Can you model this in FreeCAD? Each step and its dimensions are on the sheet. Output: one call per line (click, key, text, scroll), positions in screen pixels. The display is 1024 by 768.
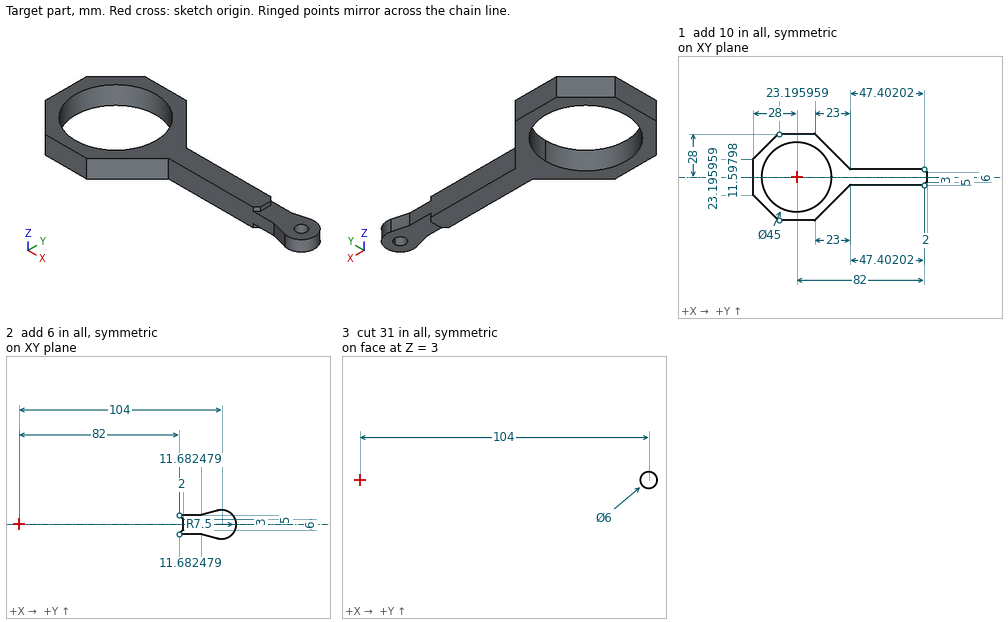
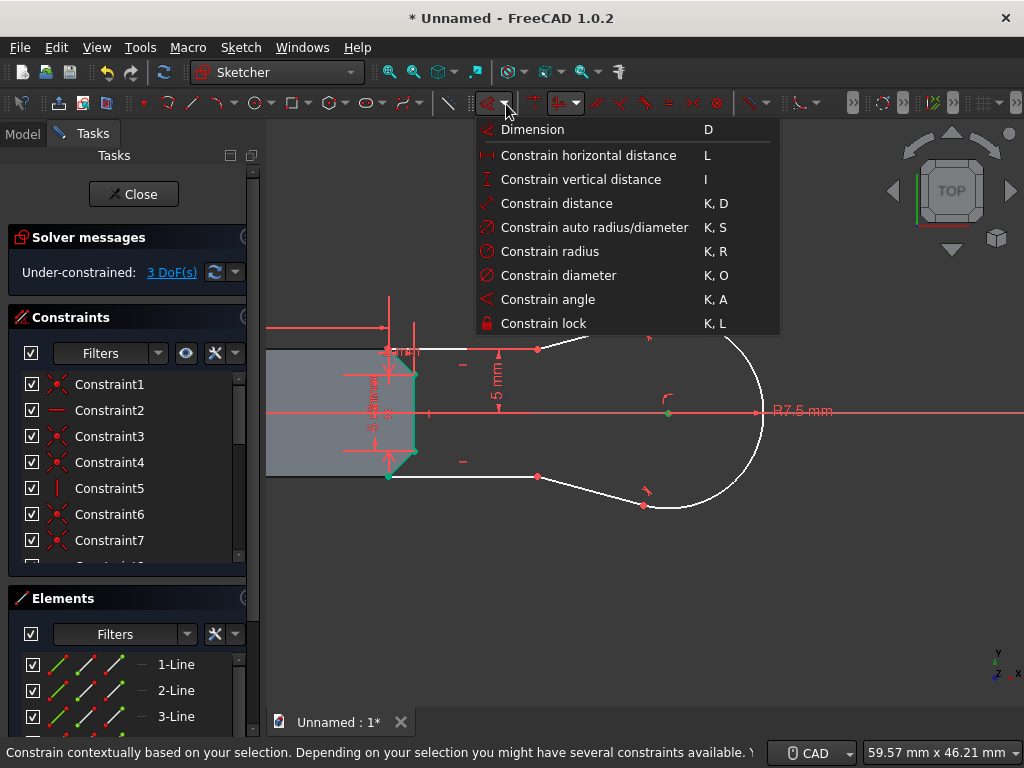
click(628, 155)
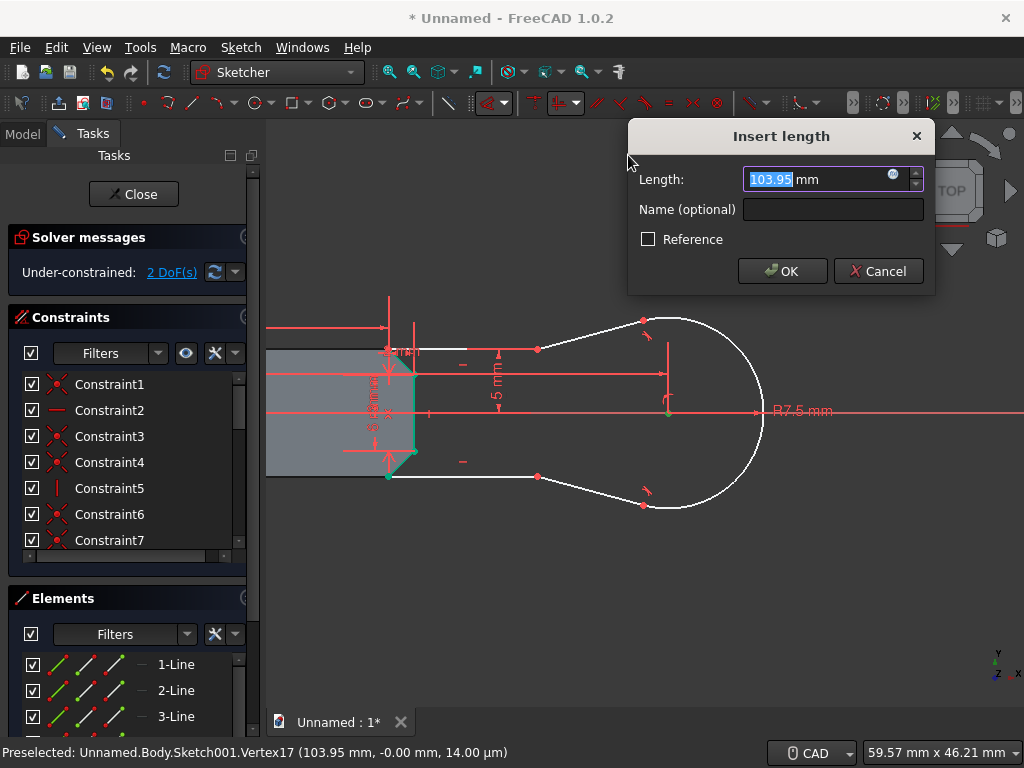
text(104)
key(Return)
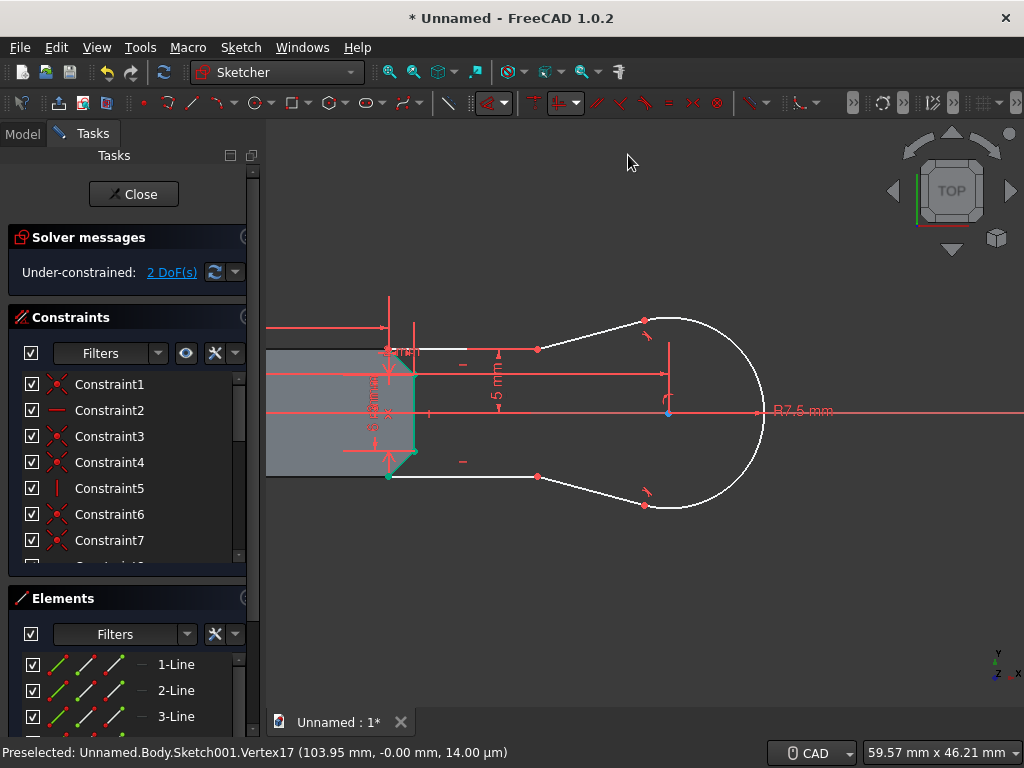
click(493, 349)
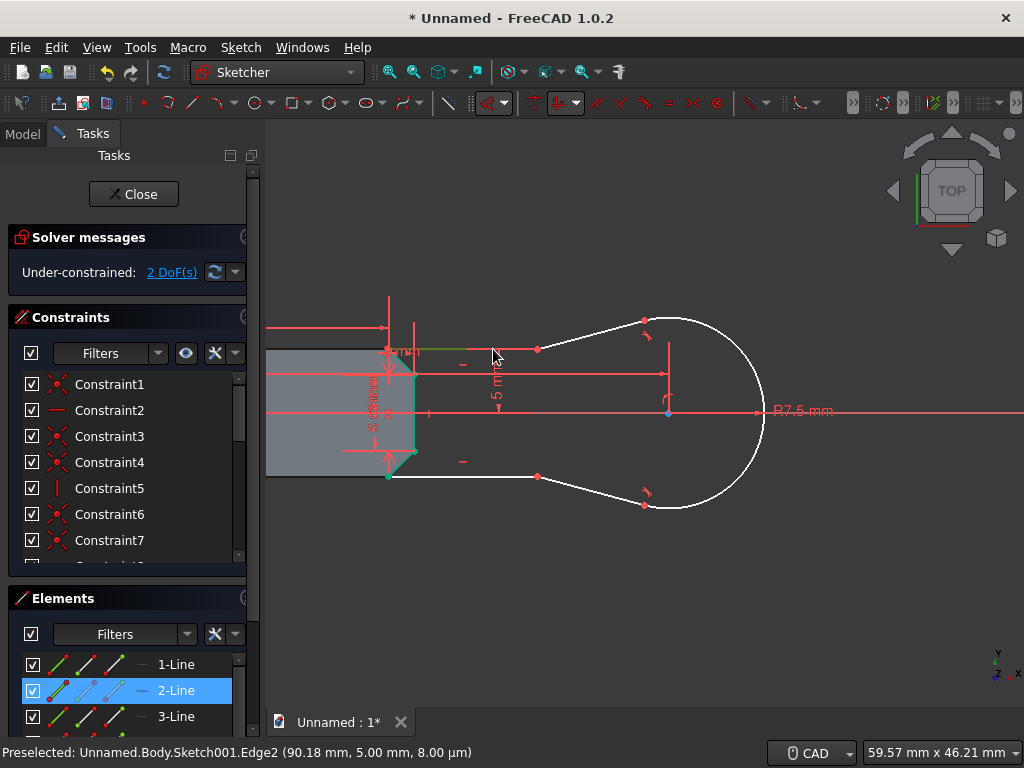
click(506, 104)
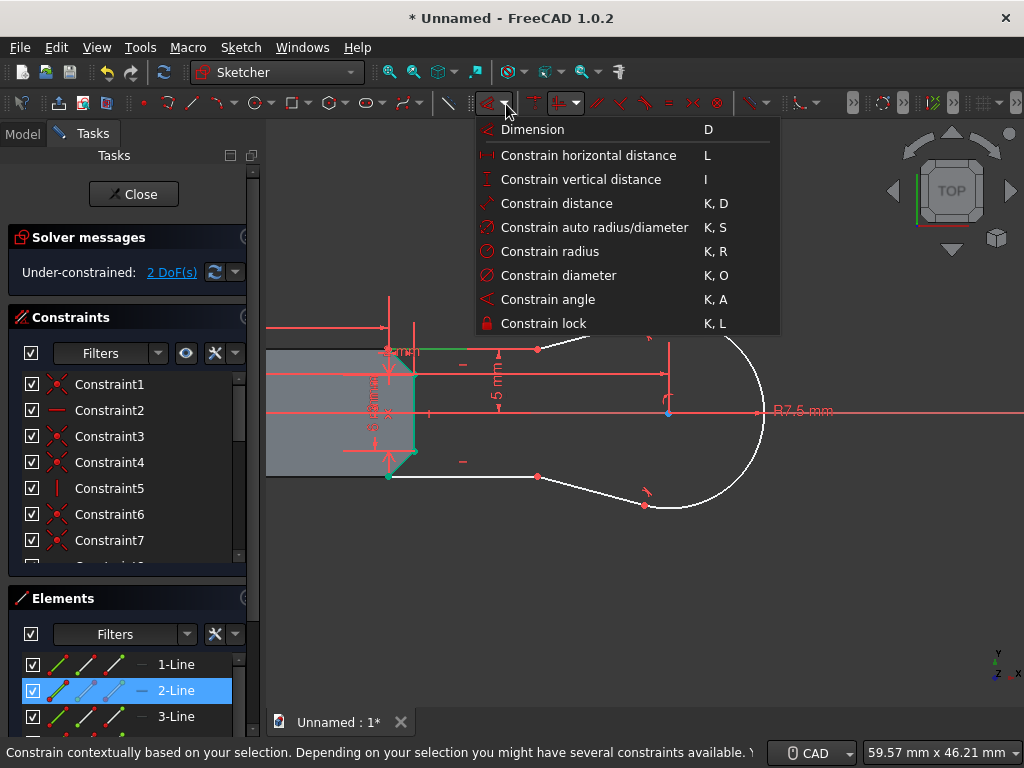
click(628, 155)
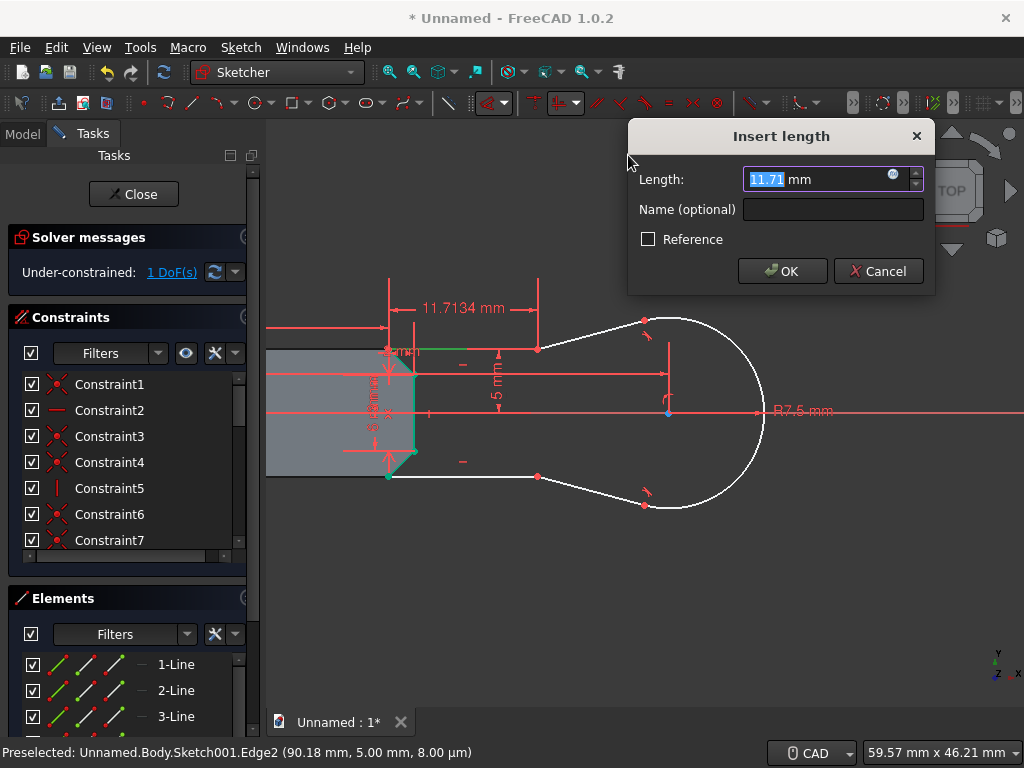
text(11.682479)
key(Return)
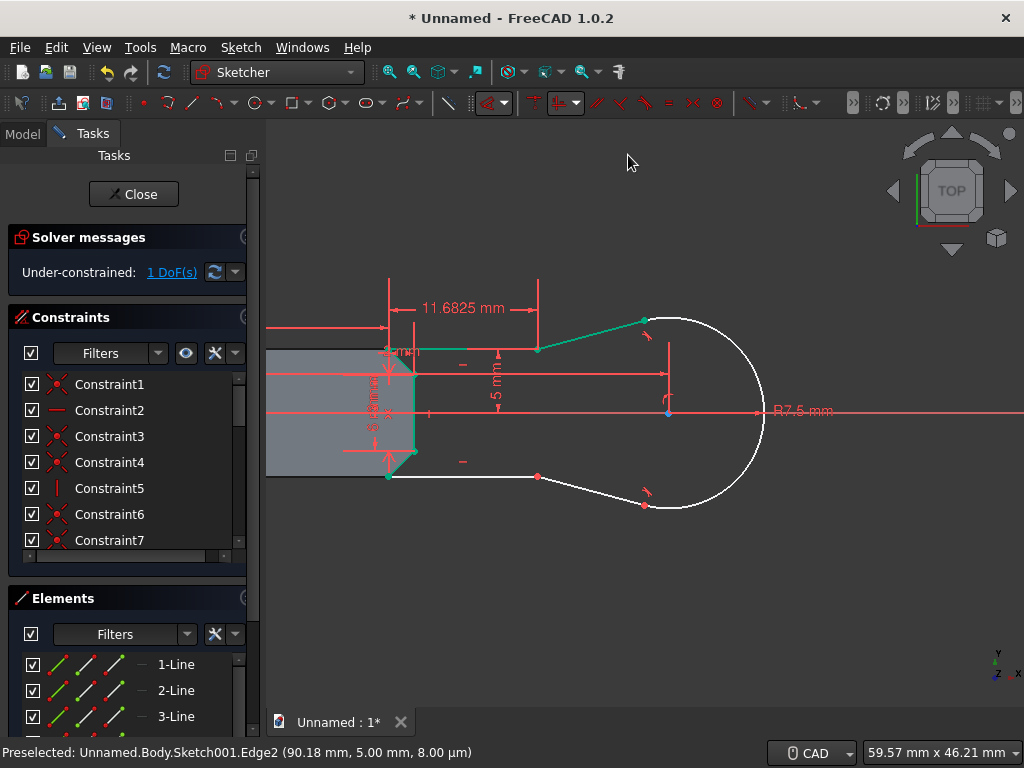
click(434, 477)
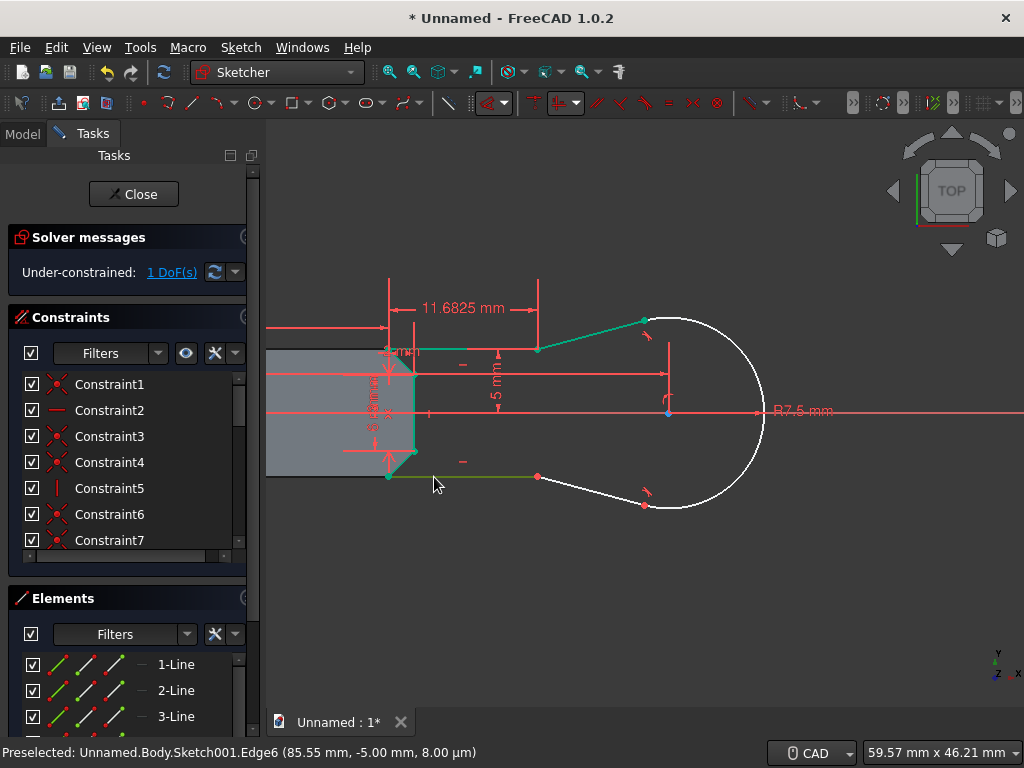
key(l)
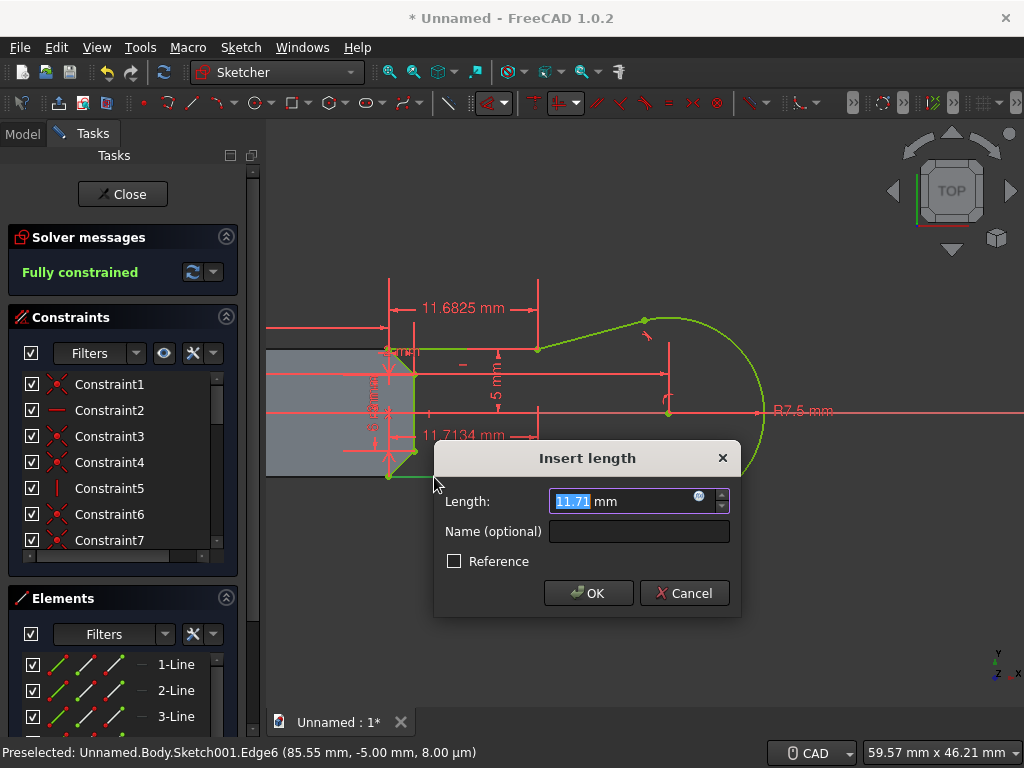
text(11.682479)
key(Return)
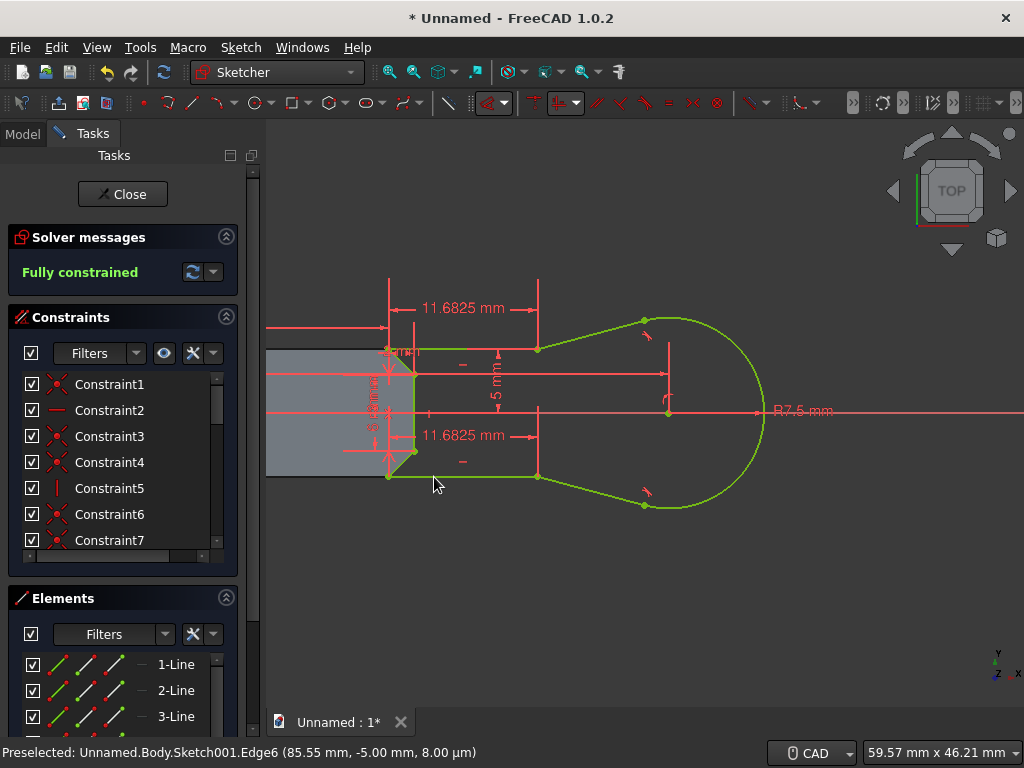
click(123, 194)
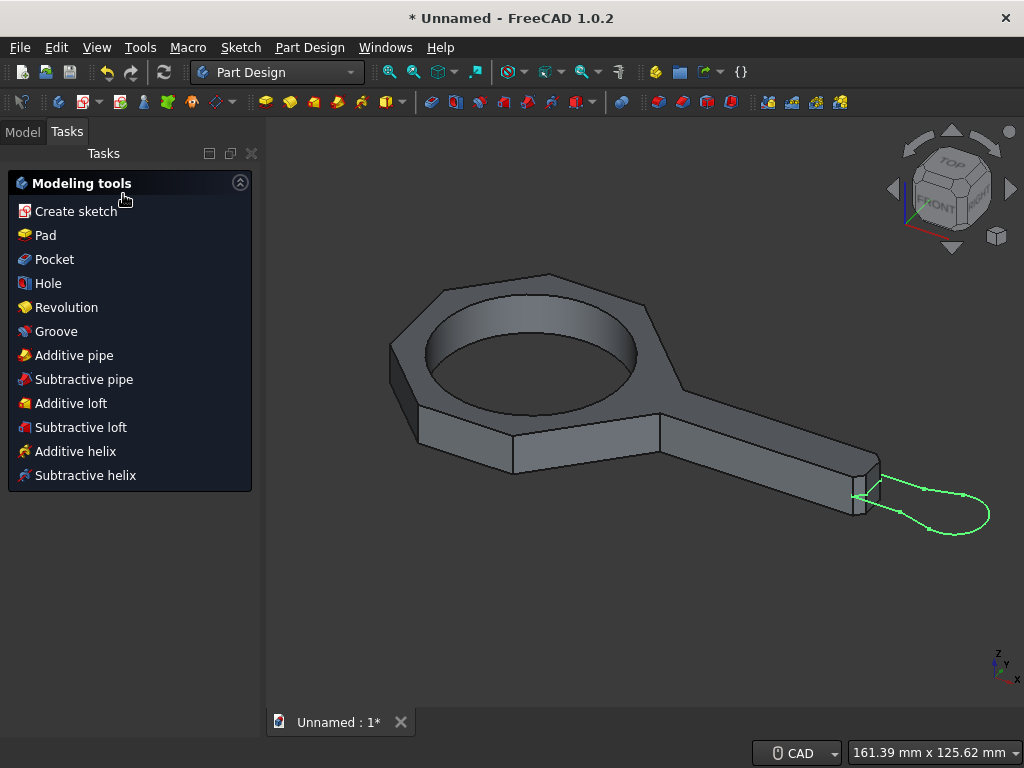
click(266, 102)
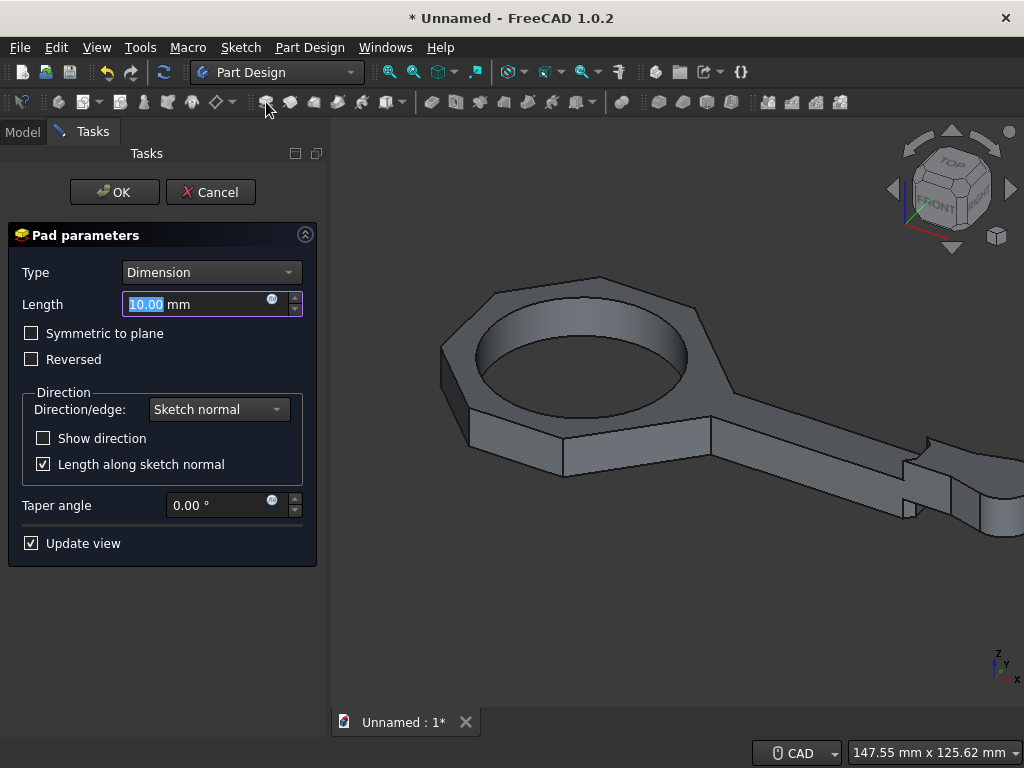
text(6)
key(Tab)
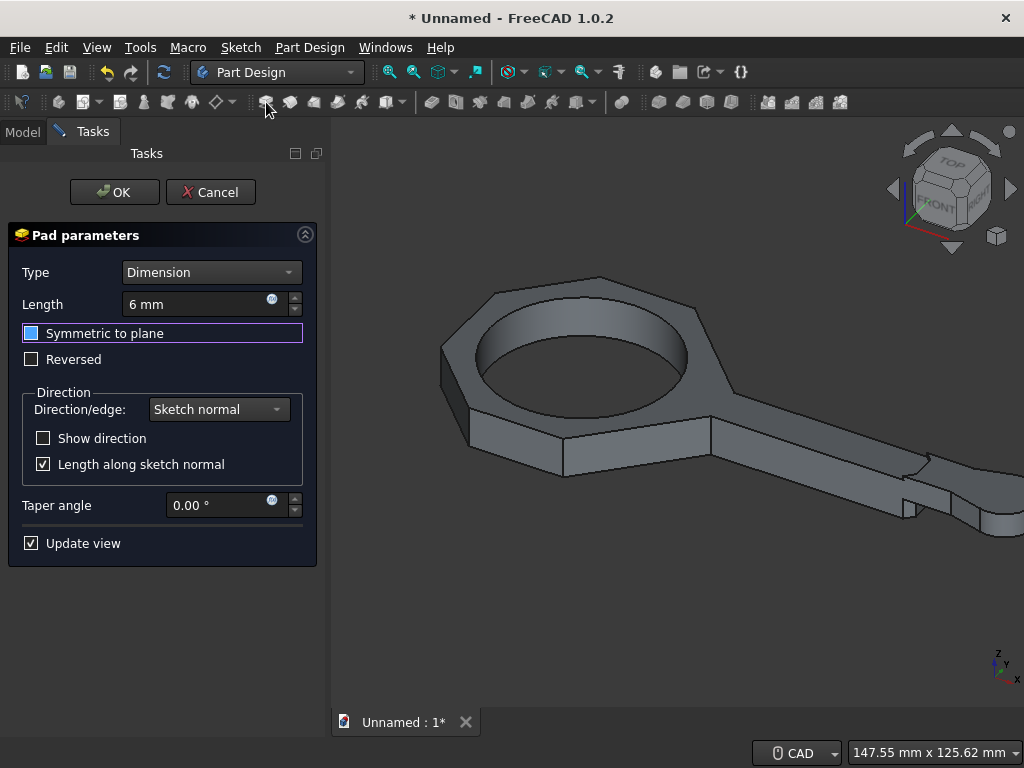
click(30, 333)